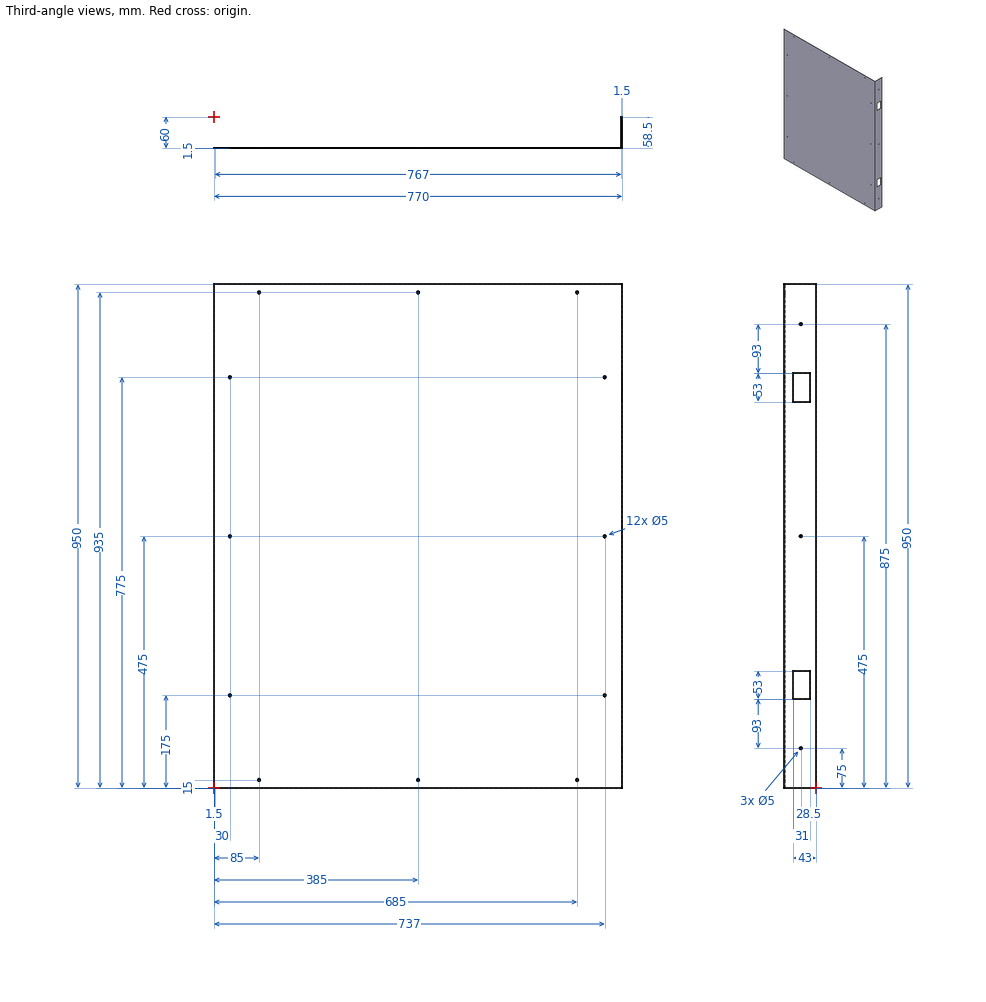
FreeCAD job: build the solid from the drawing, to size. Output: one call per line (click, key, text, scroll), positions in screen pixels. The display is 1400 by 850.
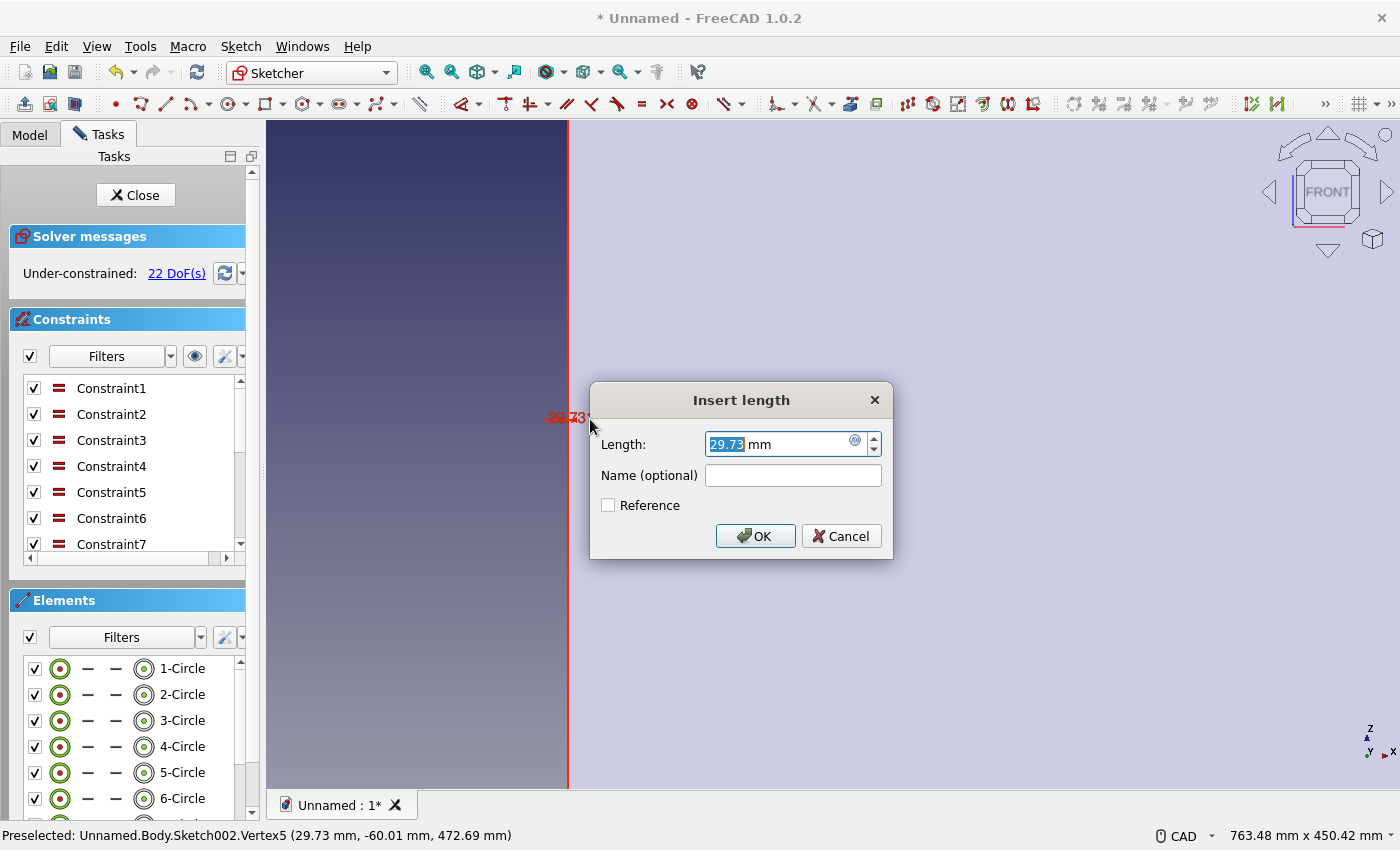
text(30)
key(Return)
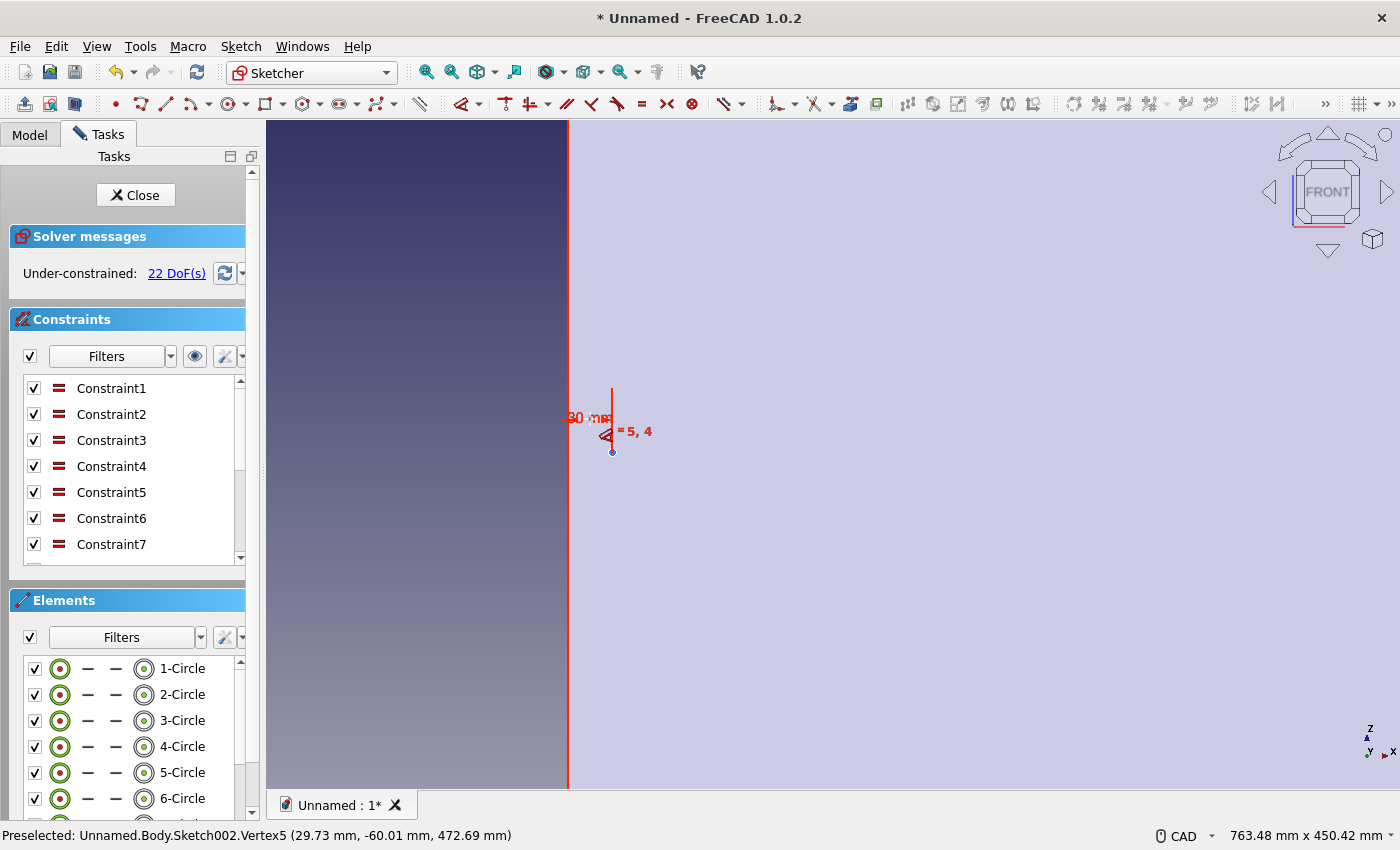
scroll(613, 453, down, 6)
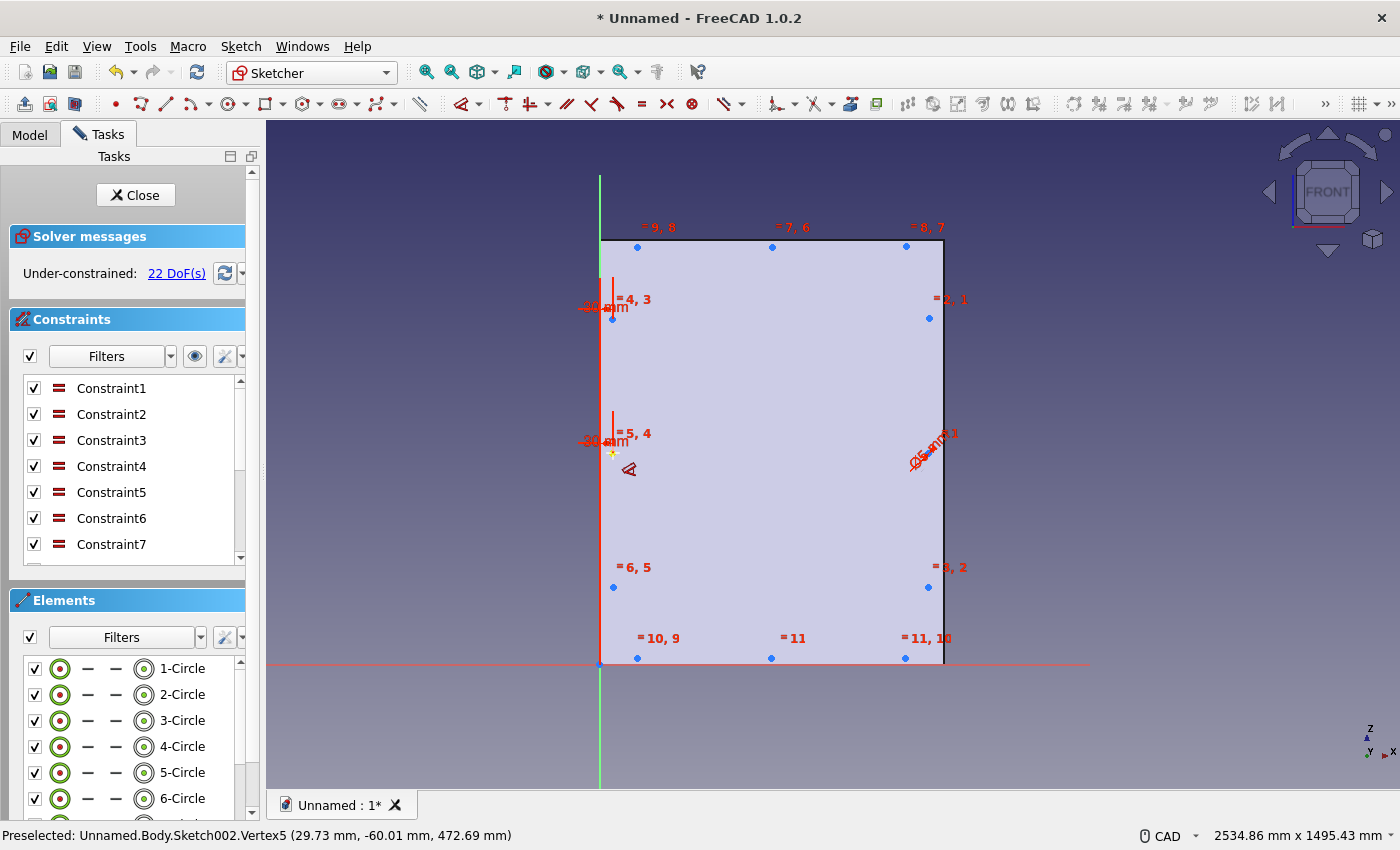
scroll(613, 587, up, 6)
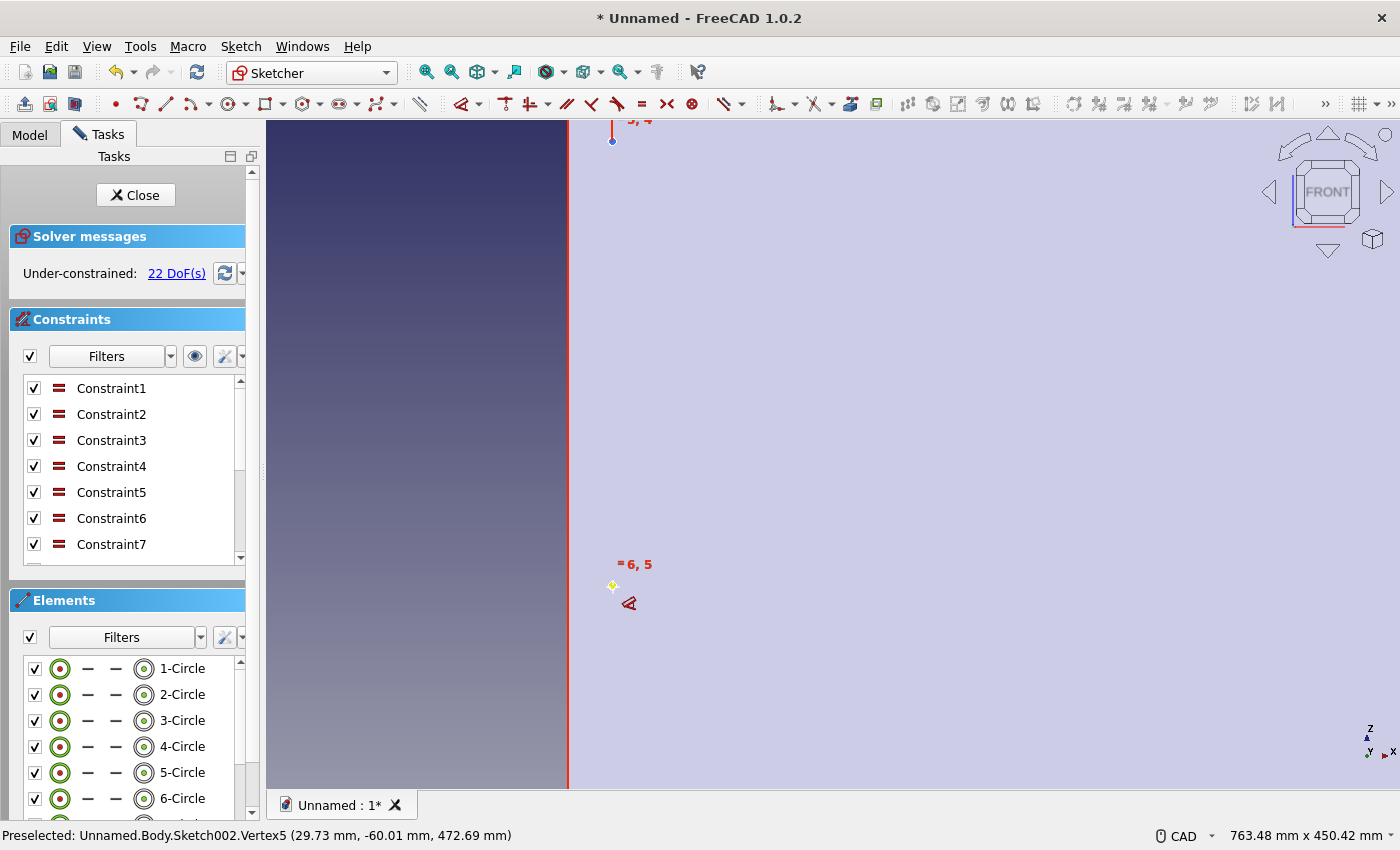
click(612, 586)
click(590, 552)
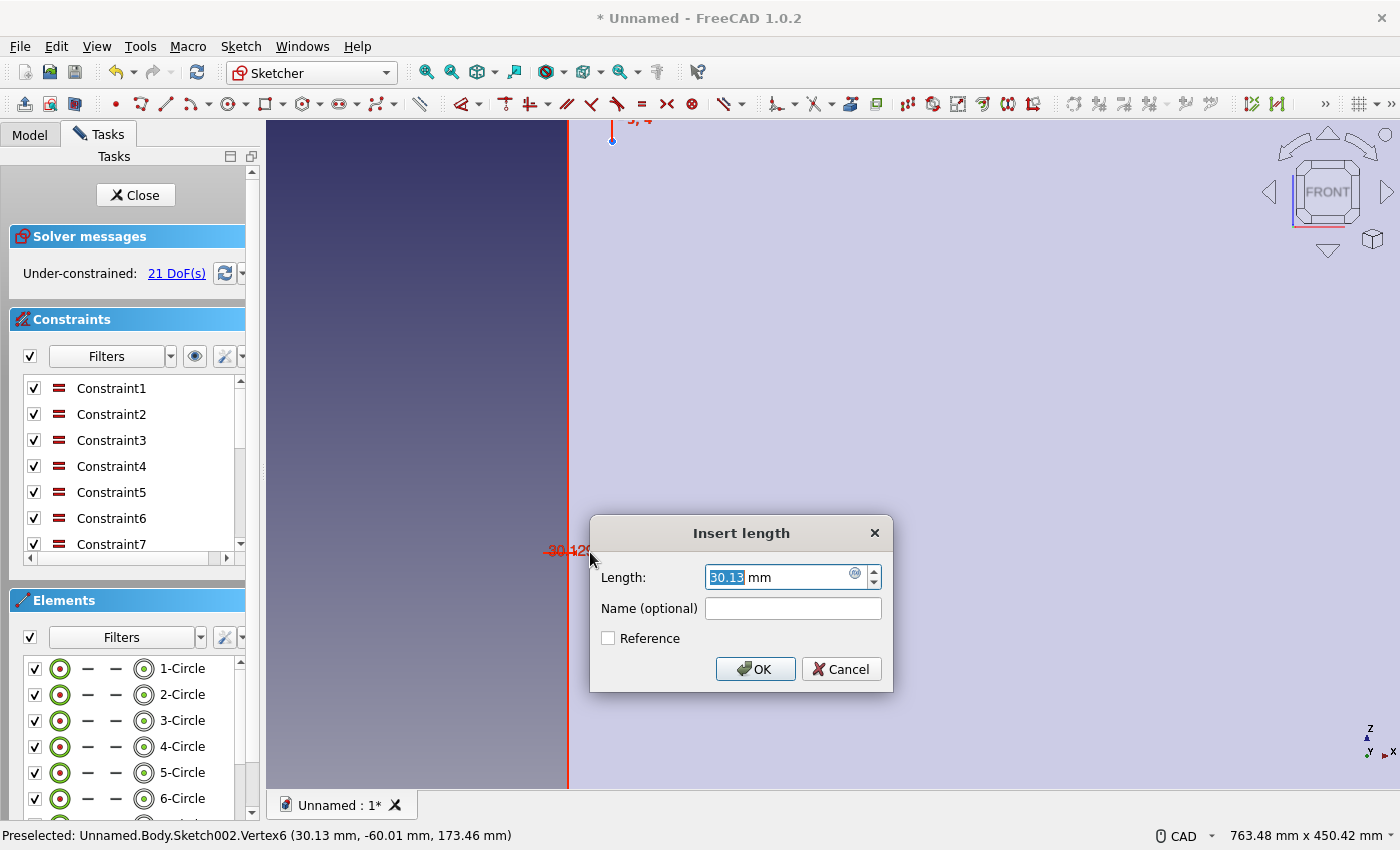
text(30)
key(Return)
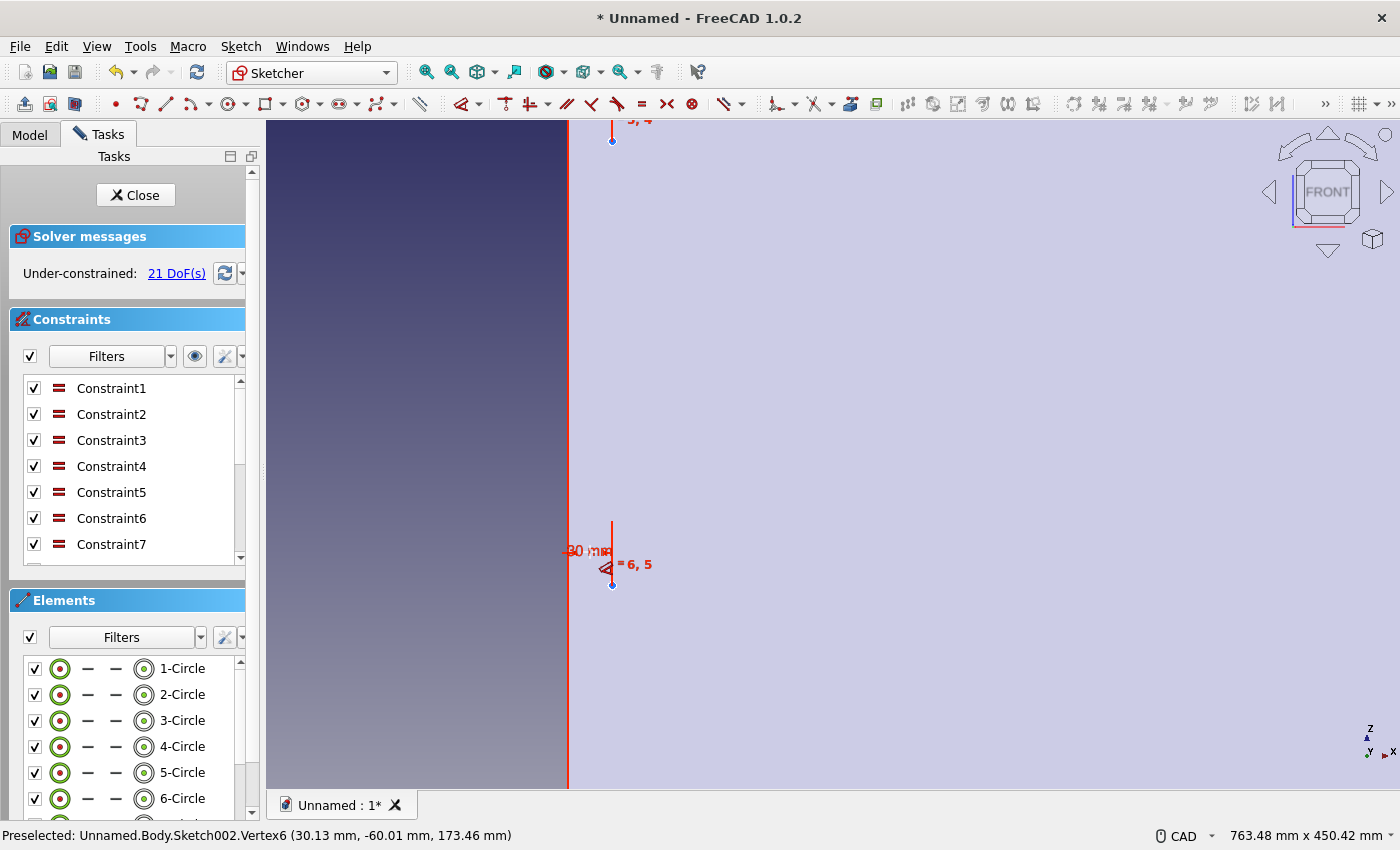
scroll(613, 587, down, 6)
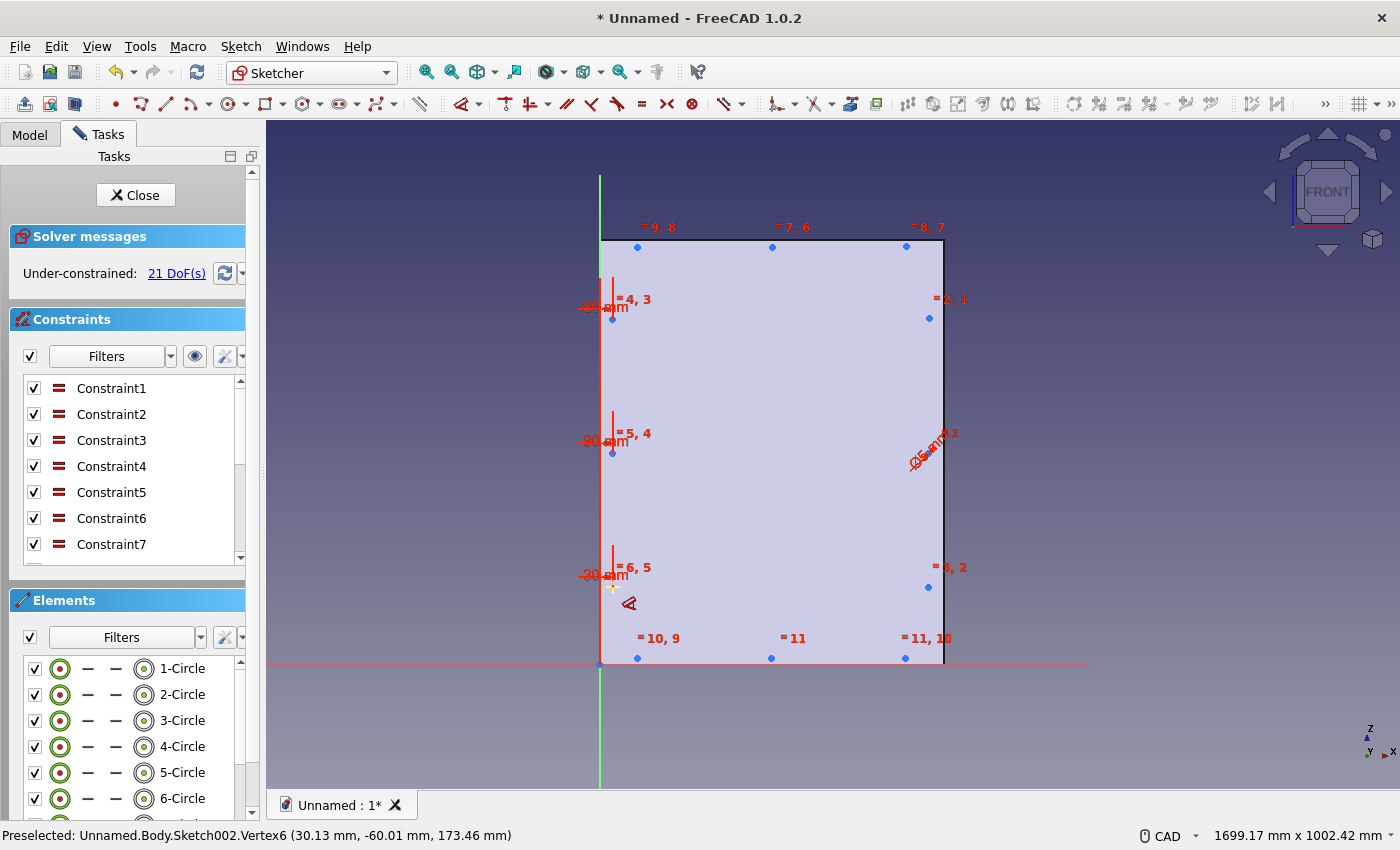
click(638, 247)
click(619, 699)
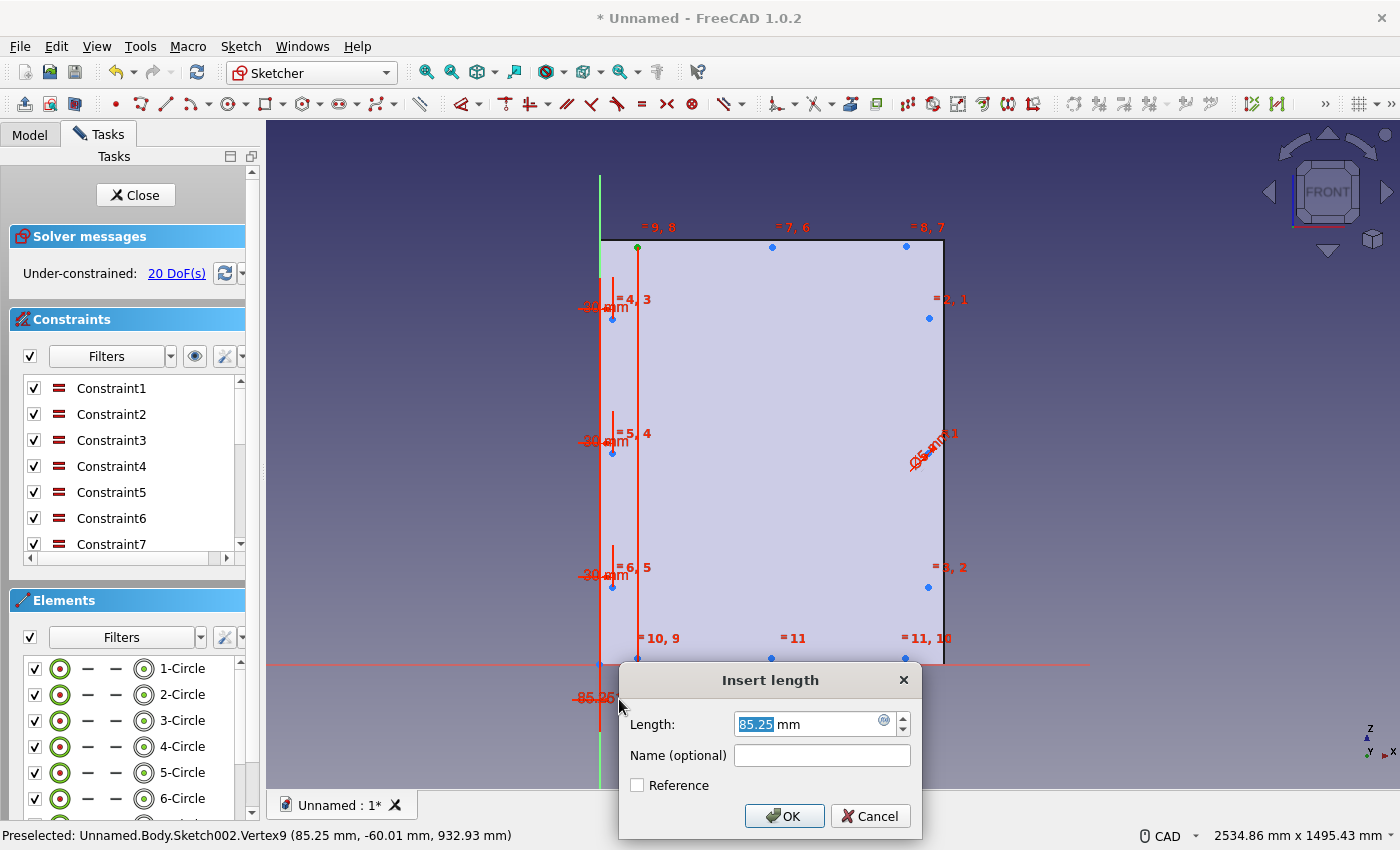
text(85)
key(Return)